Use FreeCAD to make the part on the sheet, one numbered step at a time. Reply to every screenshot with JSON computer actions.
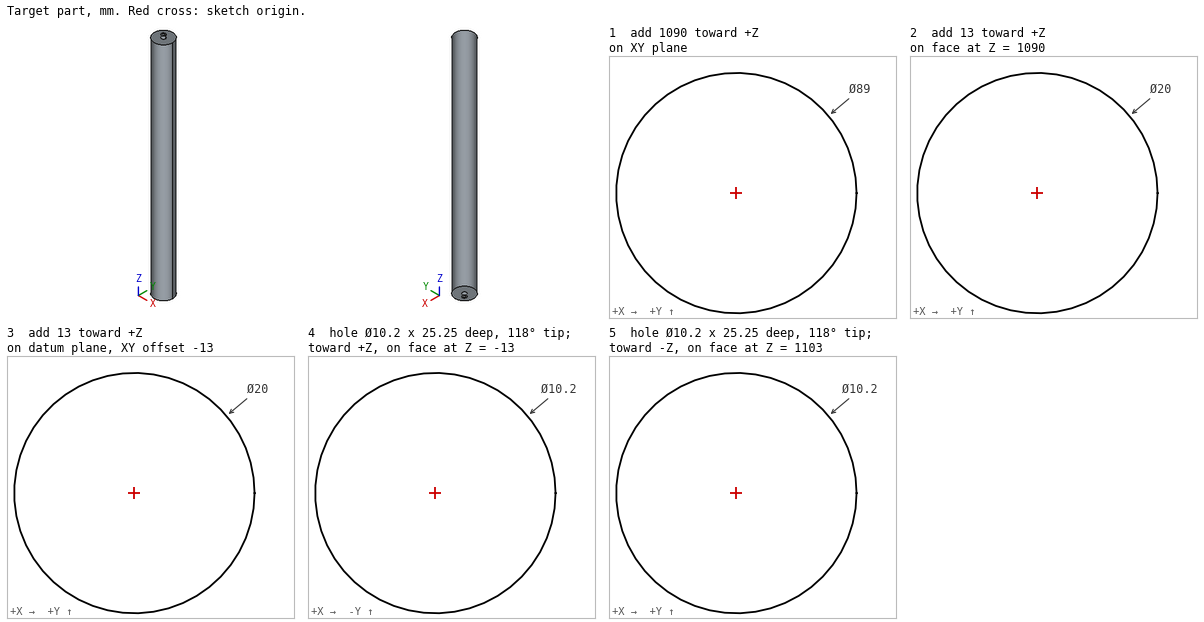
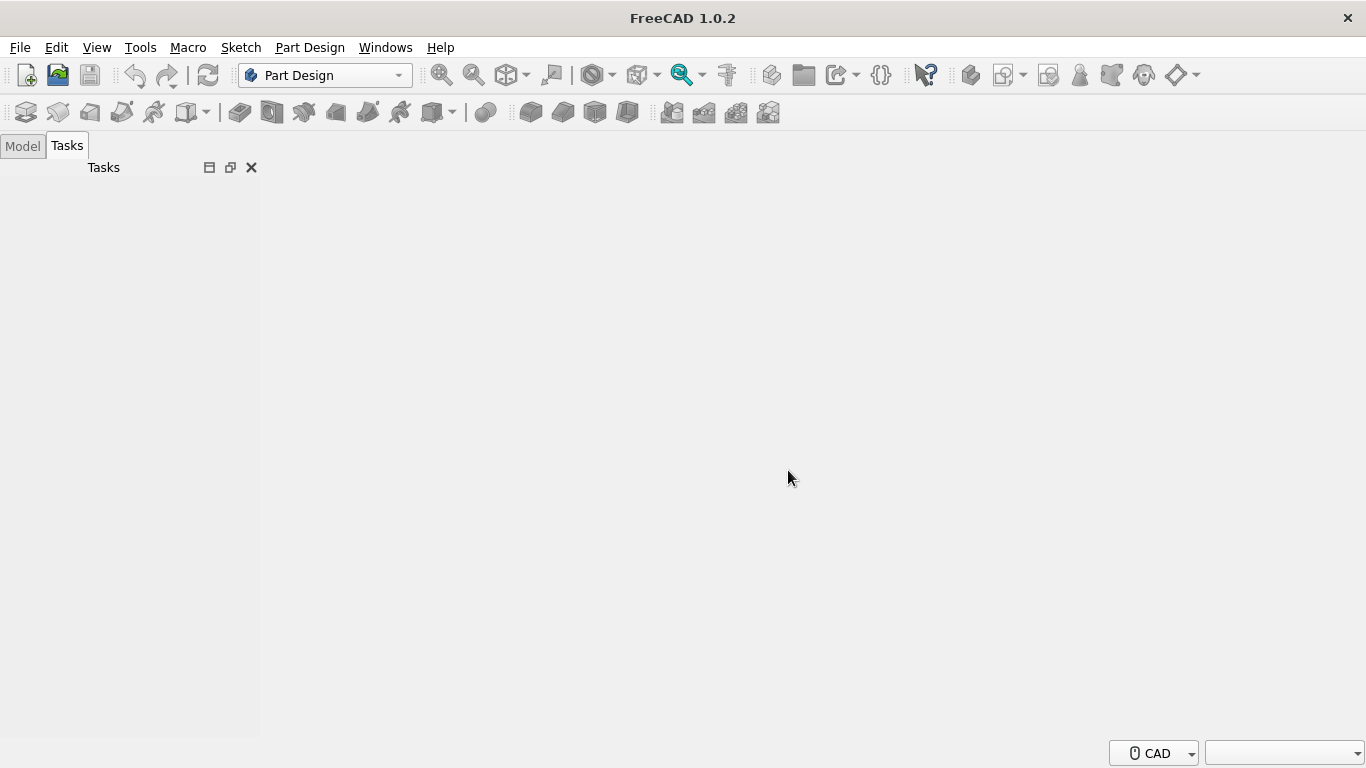
{"action": "key", "text": "ctrl+n"}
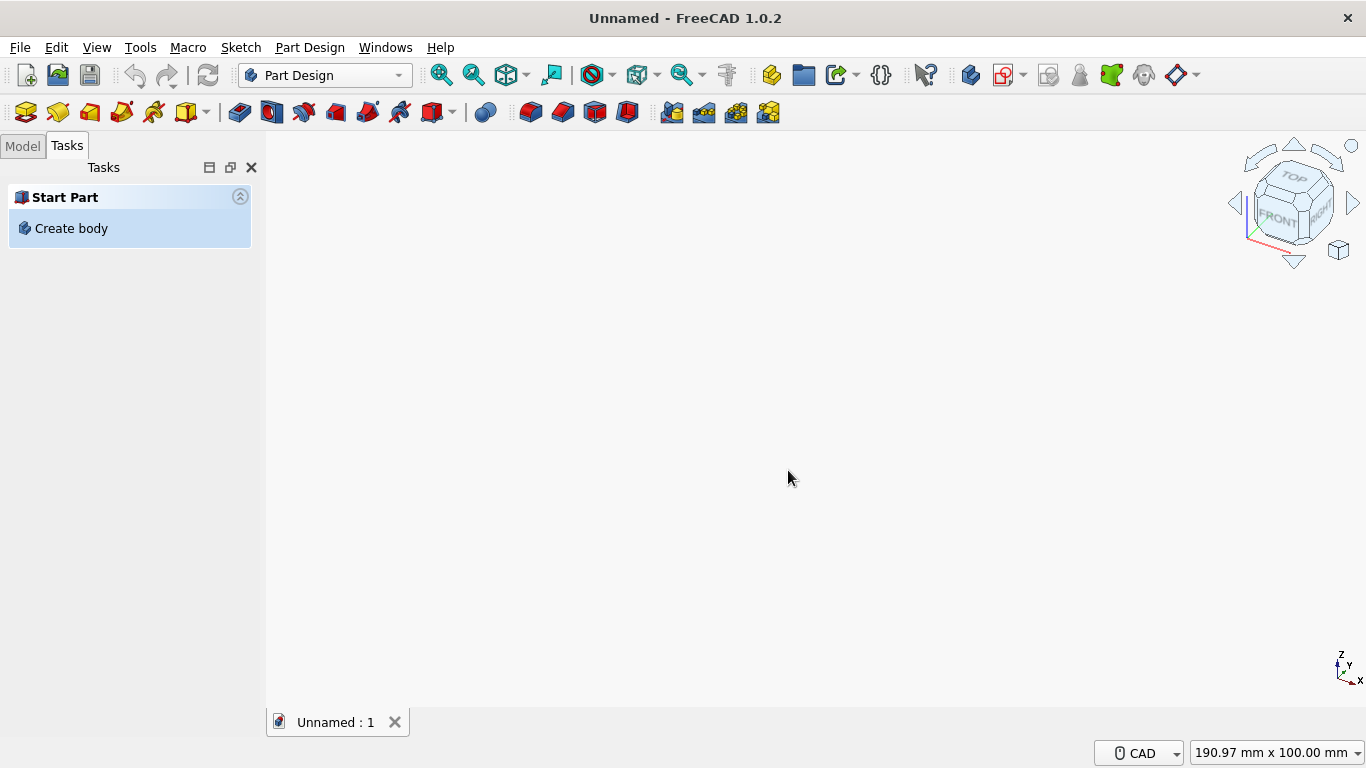
{"action": "left_click", "coordinate": [1004, 76]}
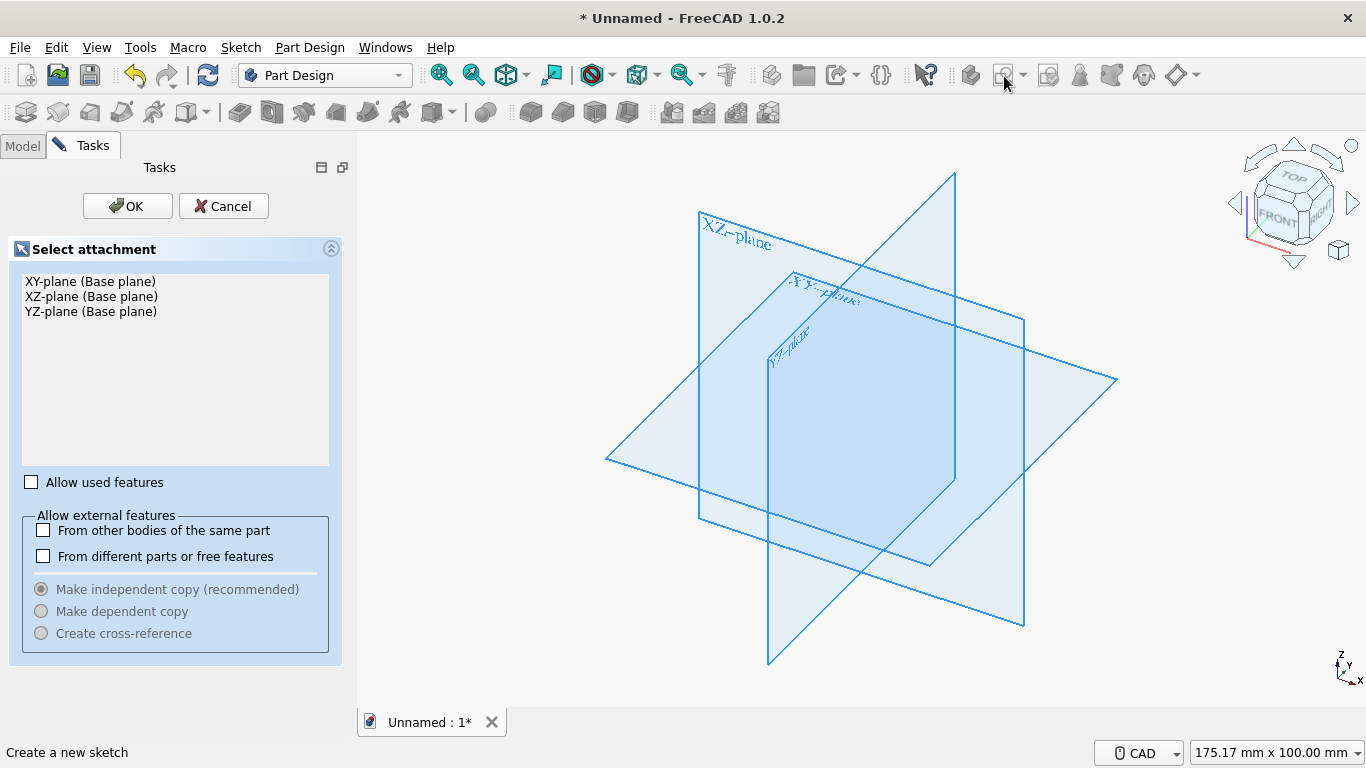
{"action": "left_click", "coordinate": [82, 282]}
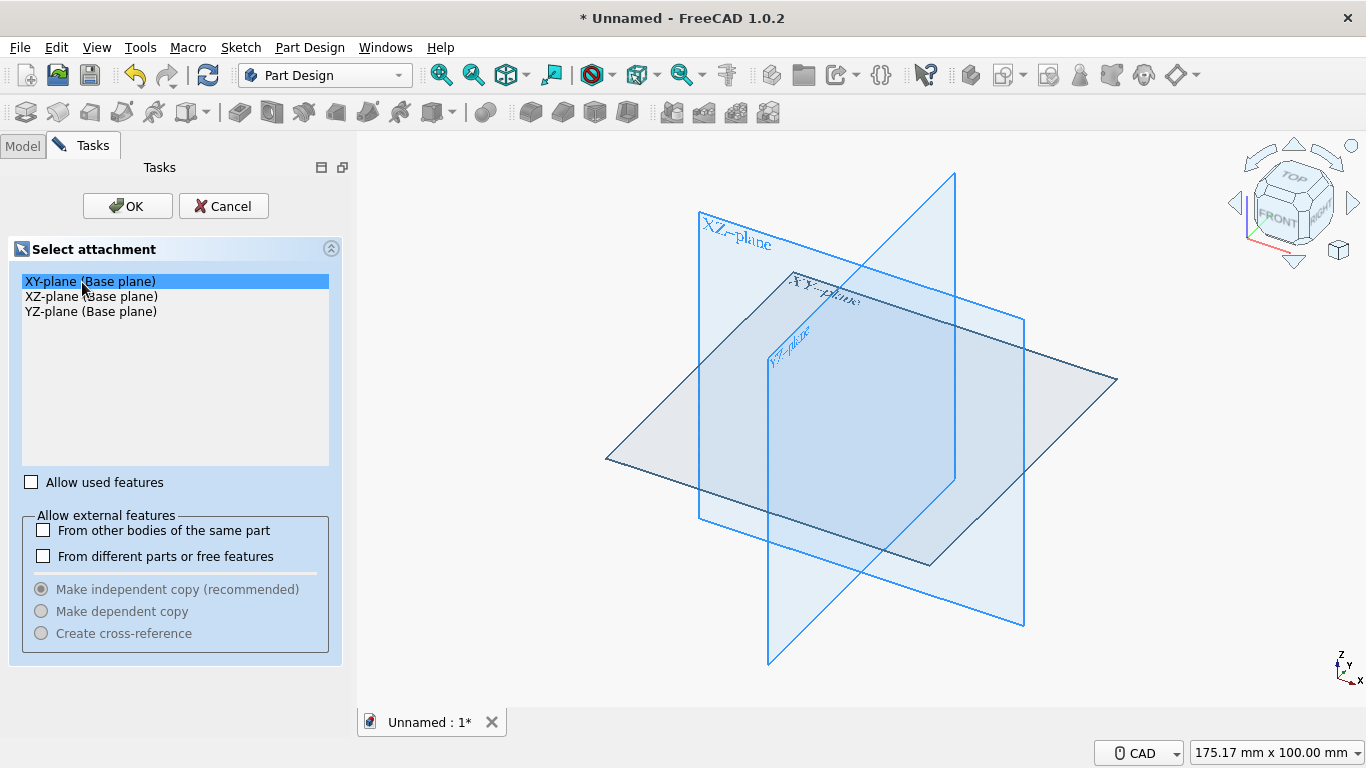
{"action": "left_click", "coordinate": [128, 206]}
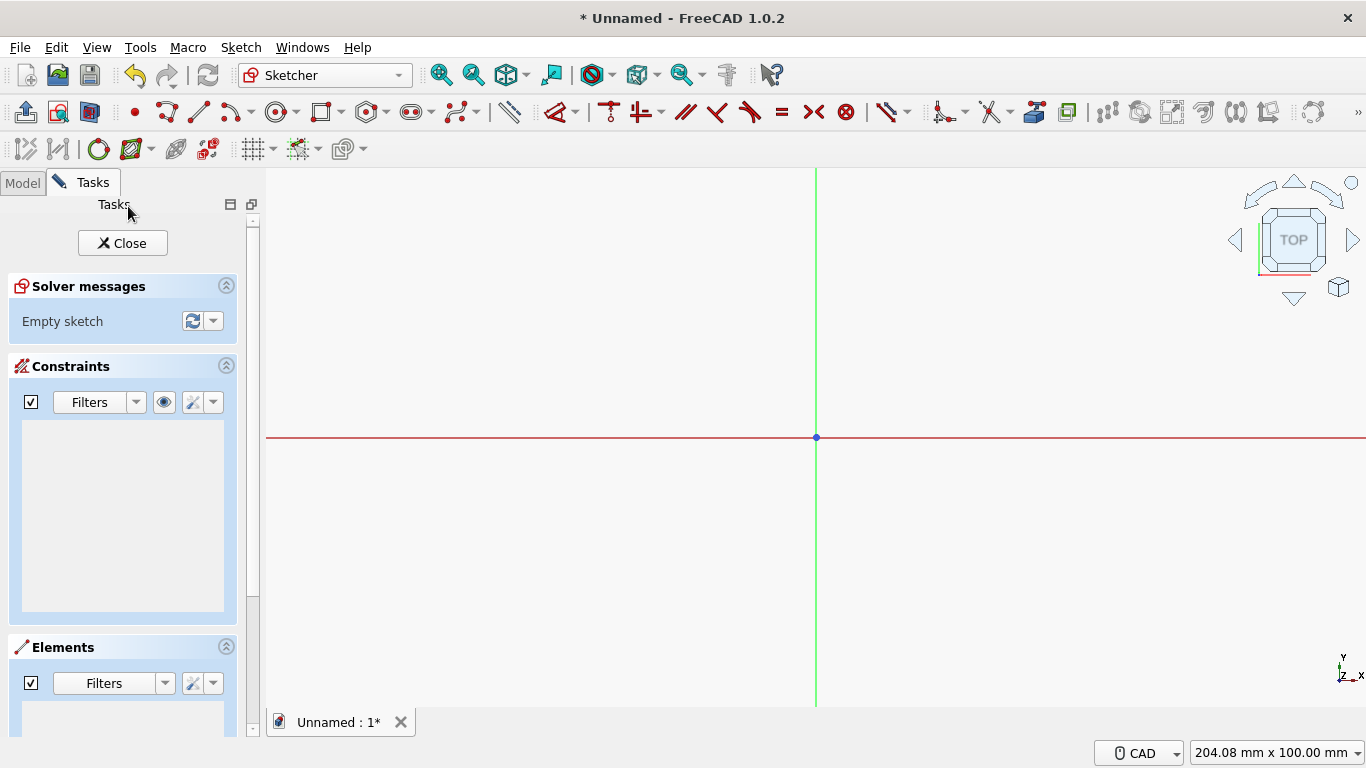
{"action": "scroll", "coordinate": [608, 438], "scroll_direction": "down", "scroll_amount": 2}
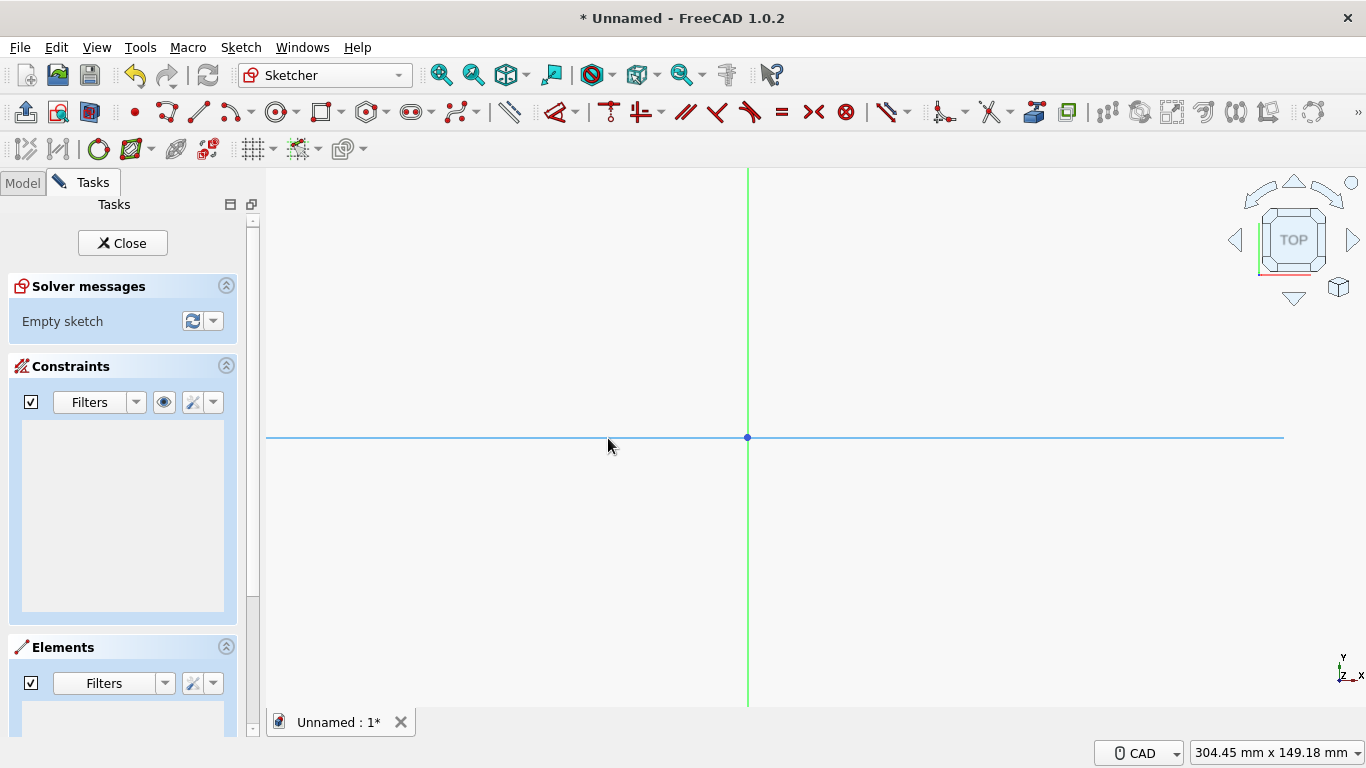
{"action": "left_click", "coordinate": [276, 112]}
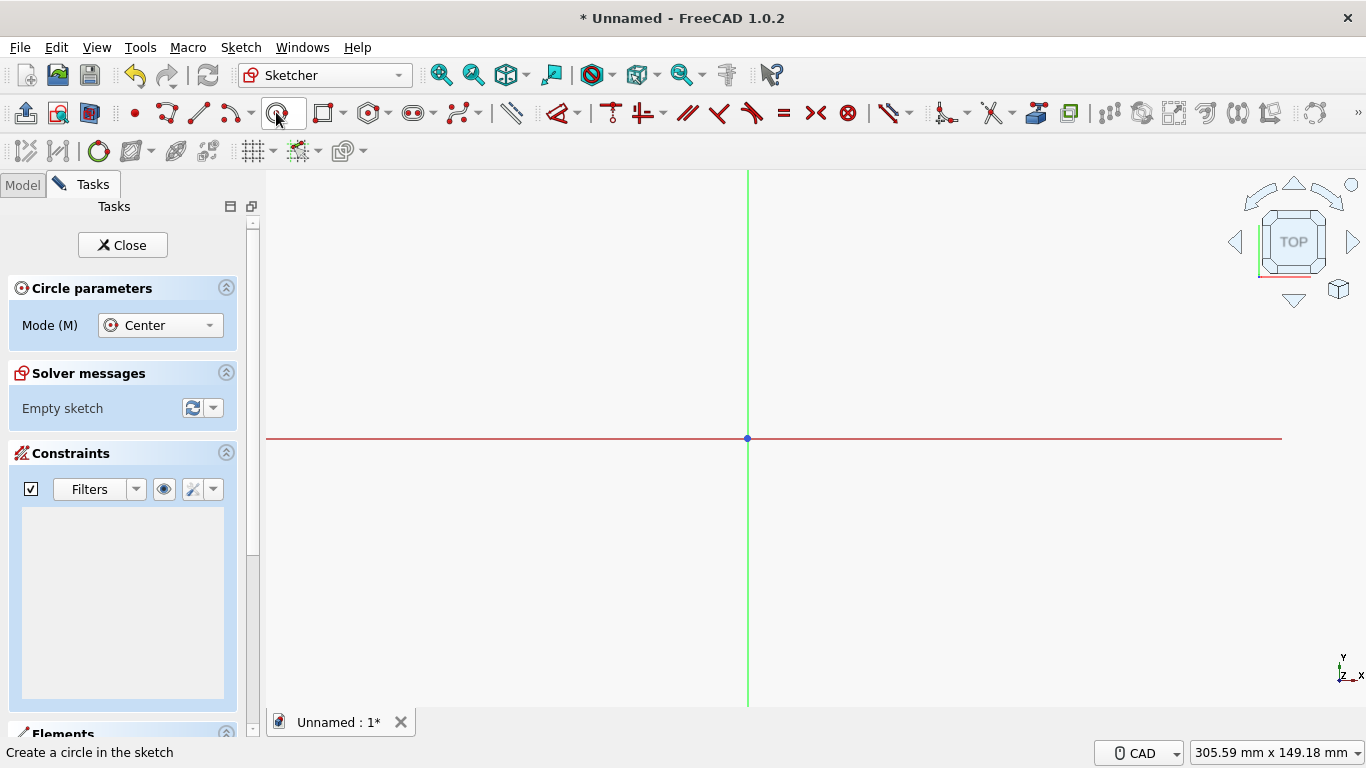
{"action": "left_click", "coordinate": [748, 439]}
{"action": "mouse_move", "coordinate": [861, 326]}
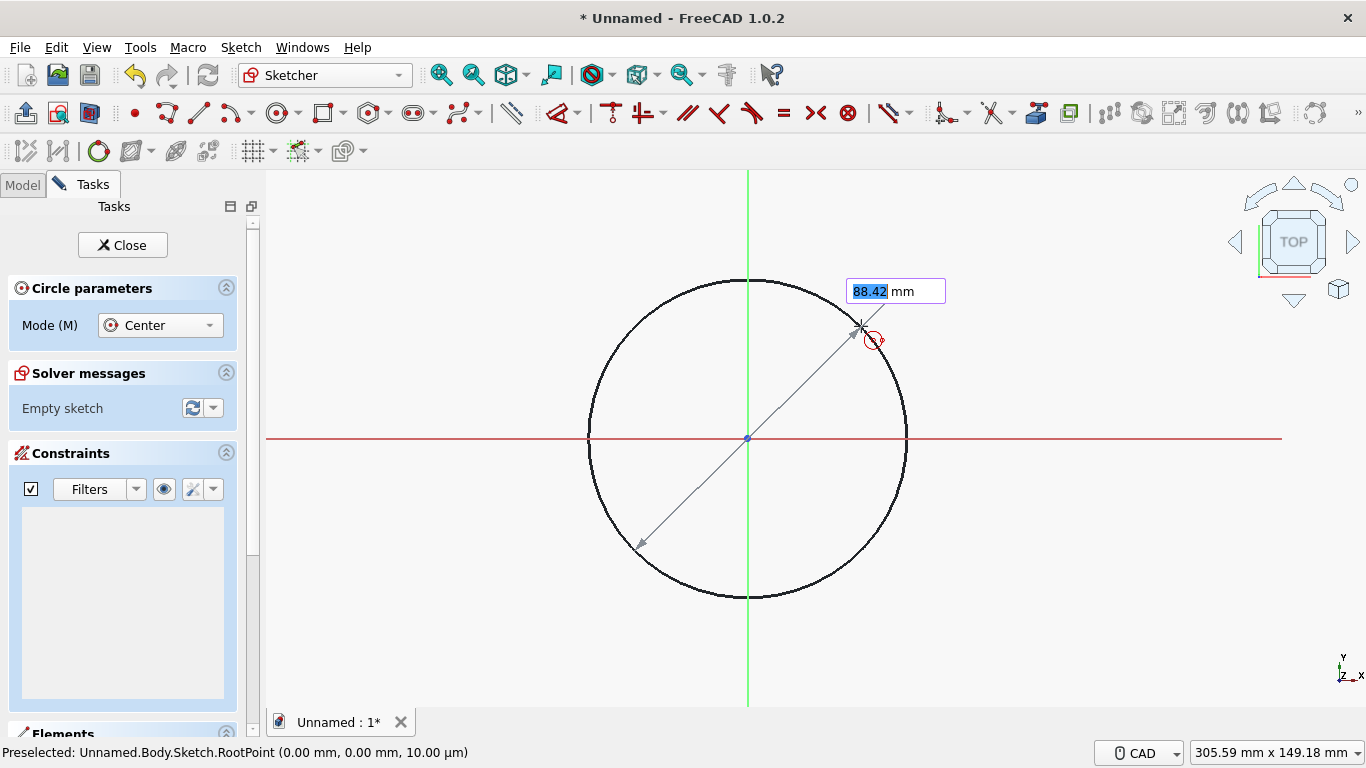
{"action": "type", "text": "89"}
{"action": "key", "text": "Return"}
{"action": "key", "text": "Escape"}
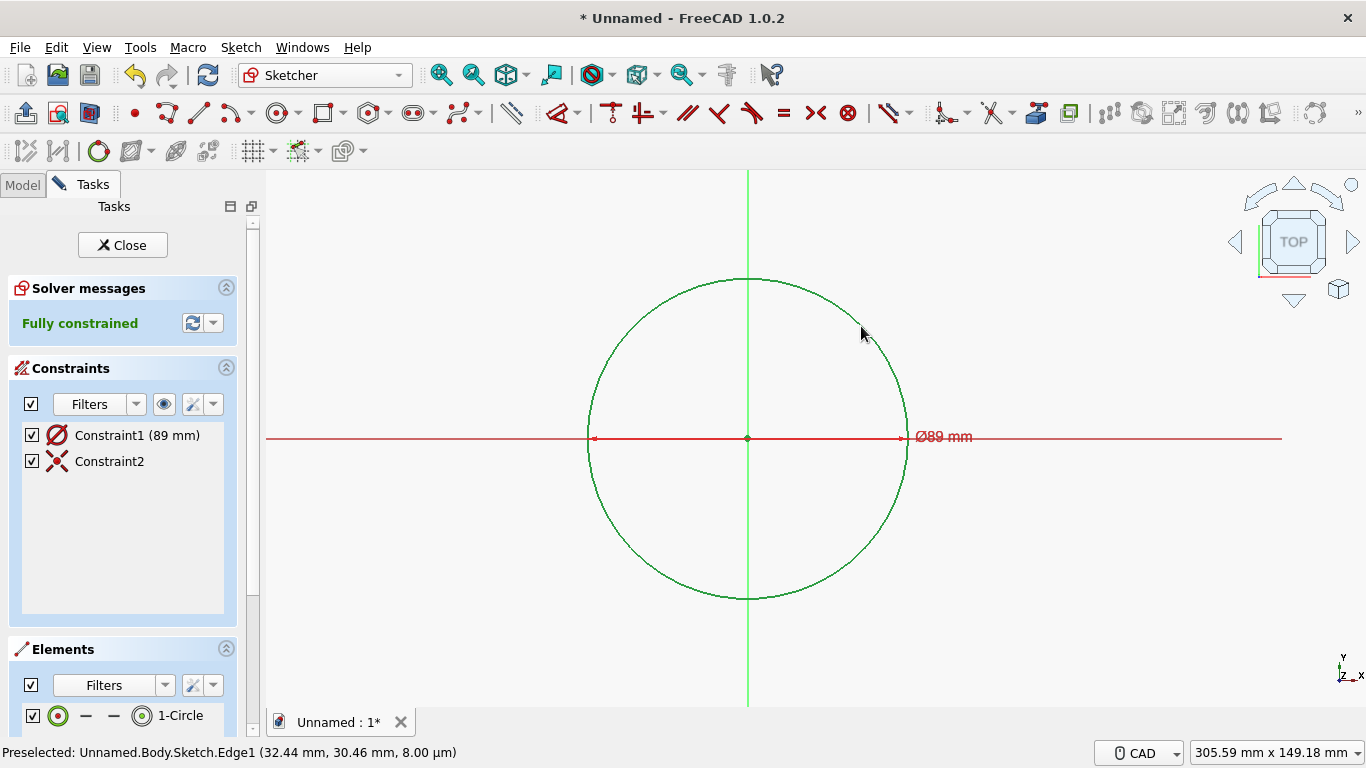
{"action": "left_click", "coordinate": [123, 245]}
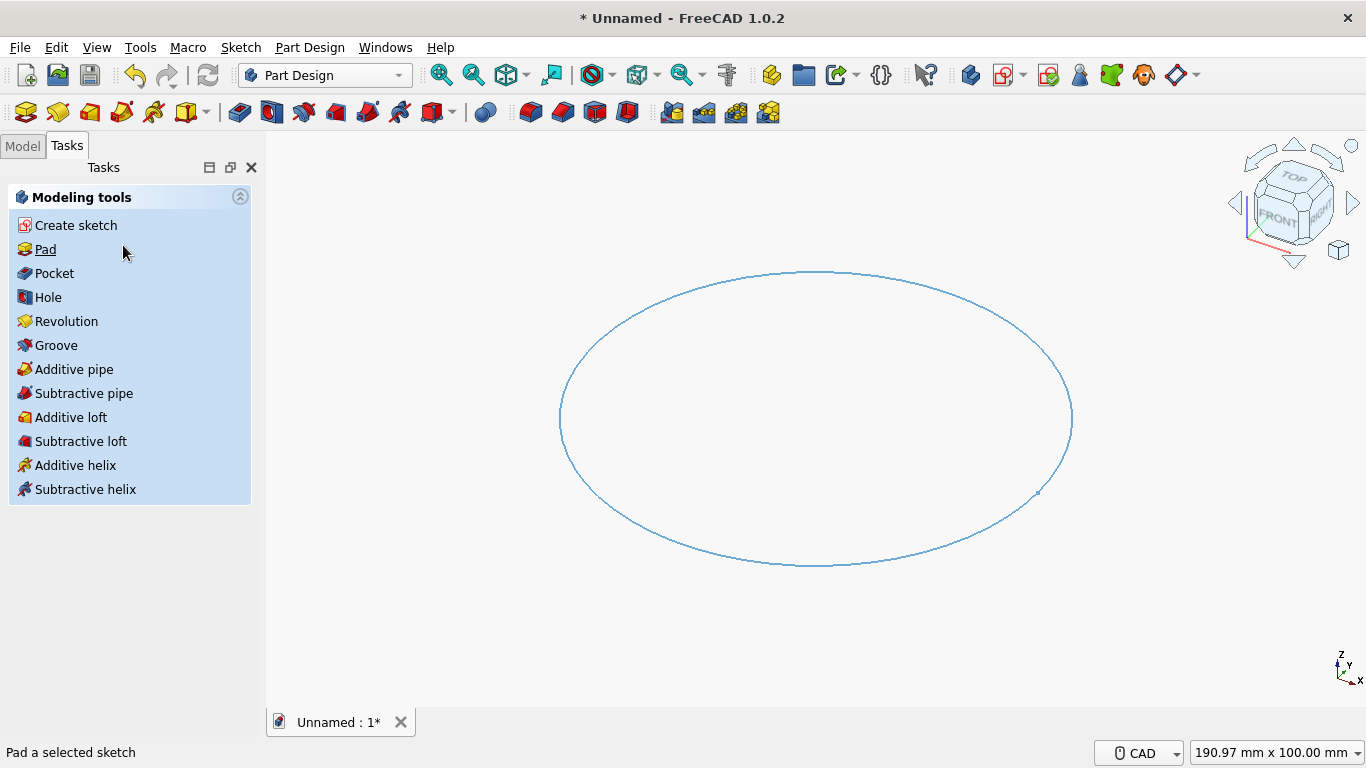
{"action": "left_click", "coordinate": [26, 112]}